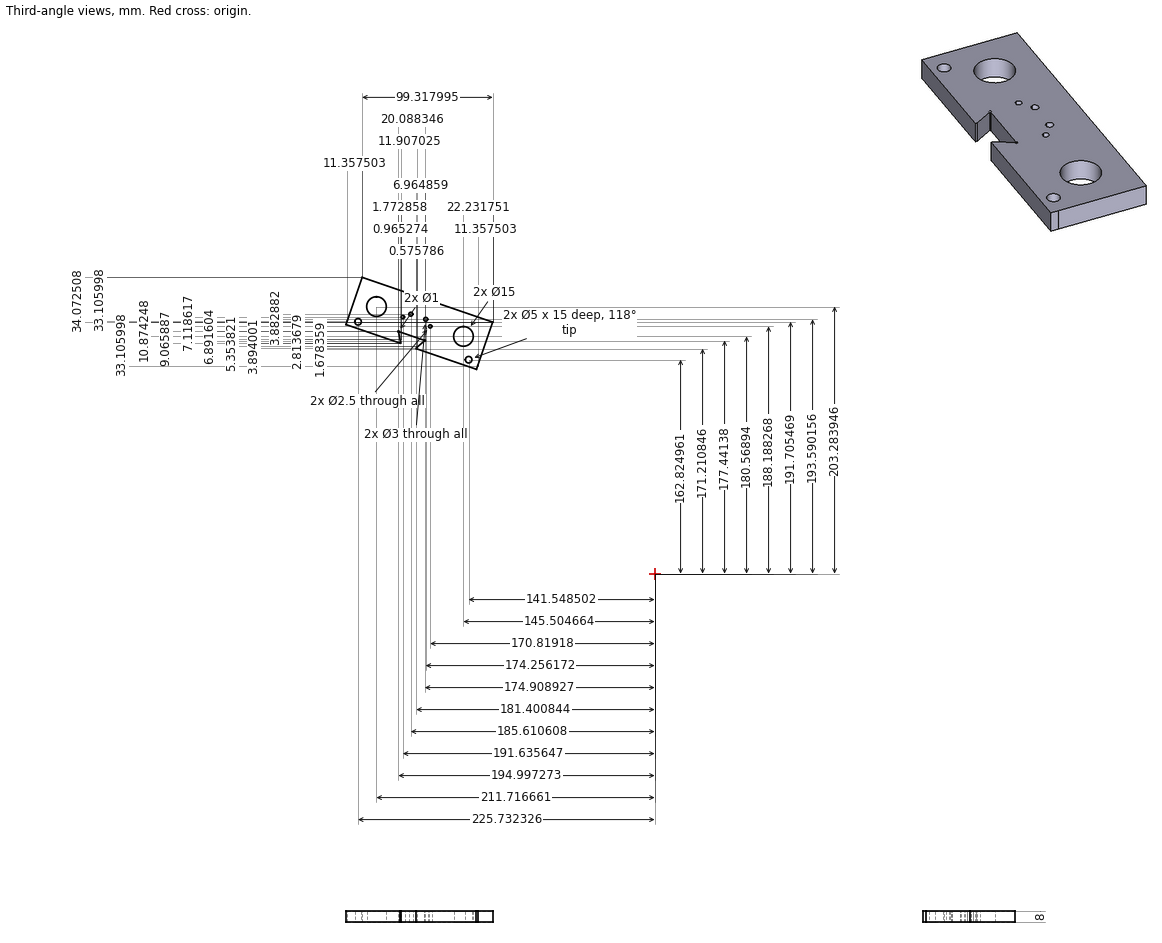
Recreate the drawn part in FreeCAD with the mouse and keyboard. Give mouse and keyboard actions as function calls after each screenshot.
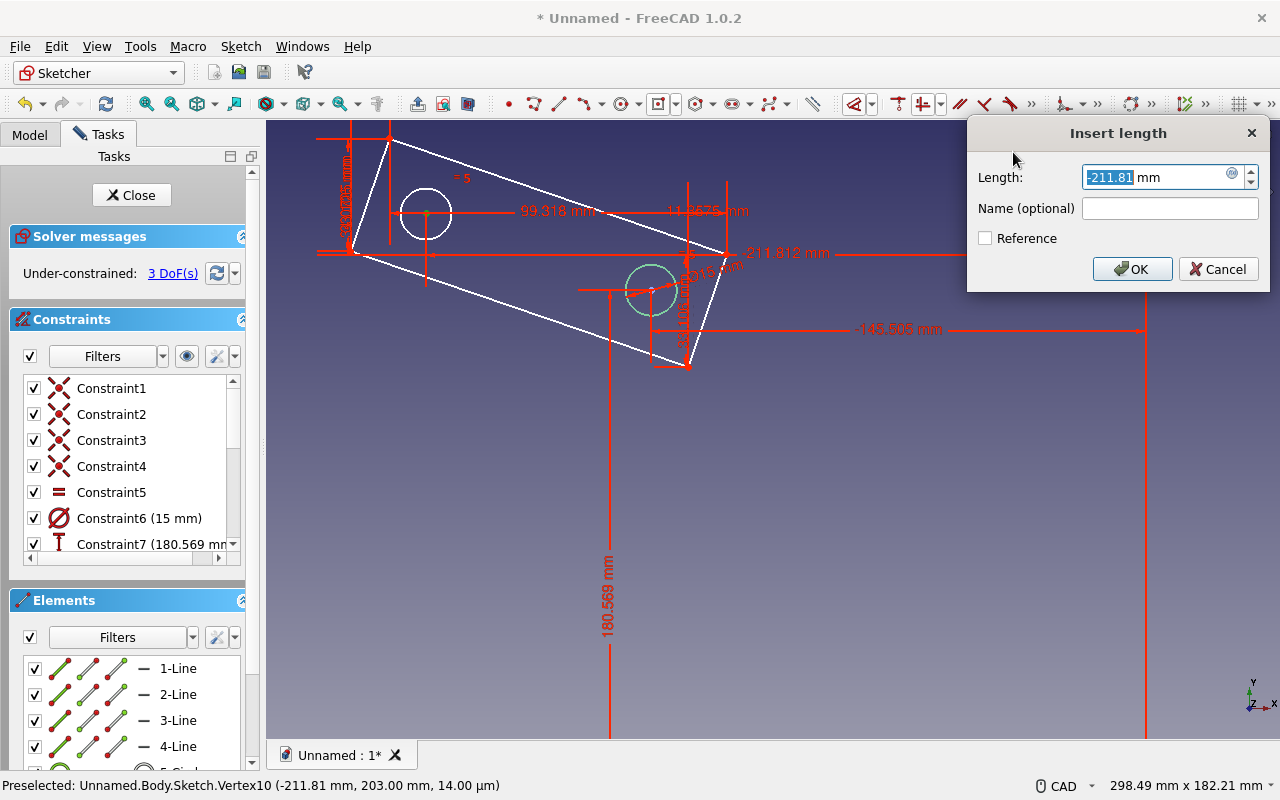
text(-211.716661)
key(Return)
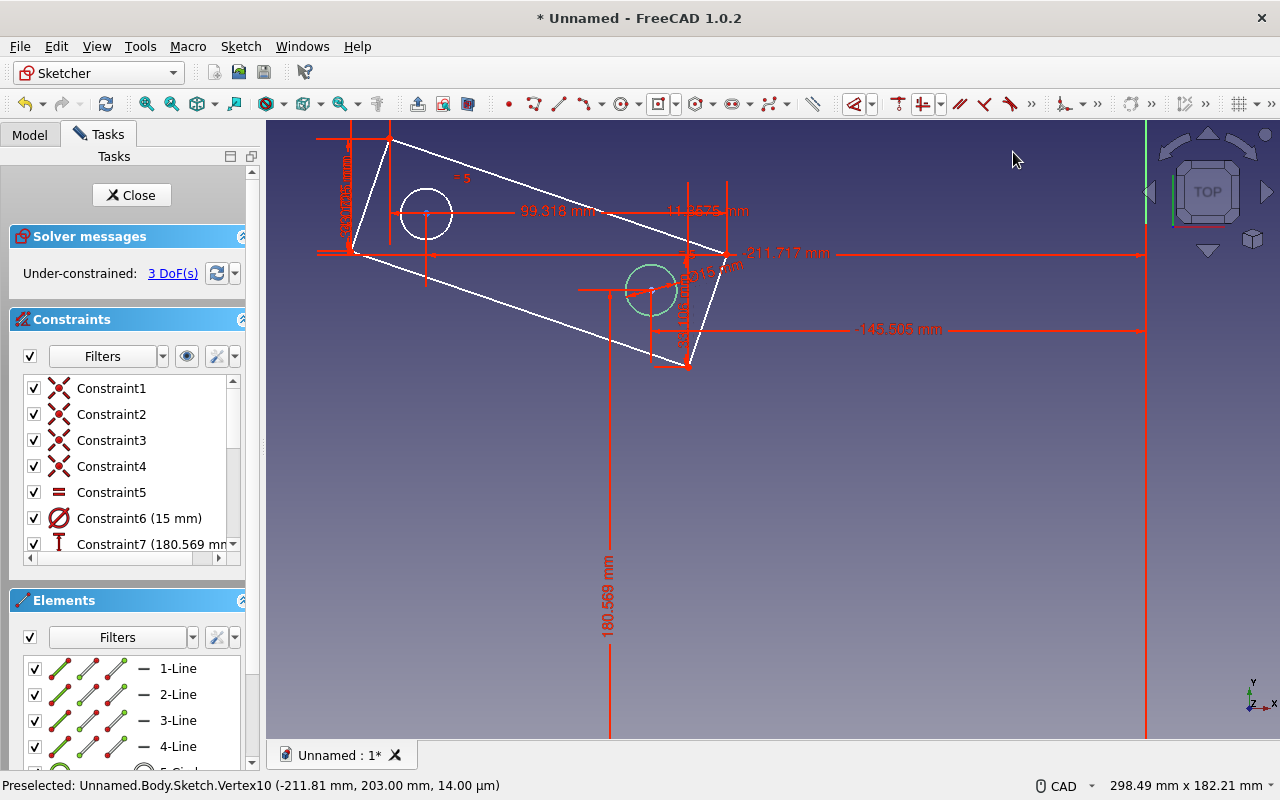
click(426, 214)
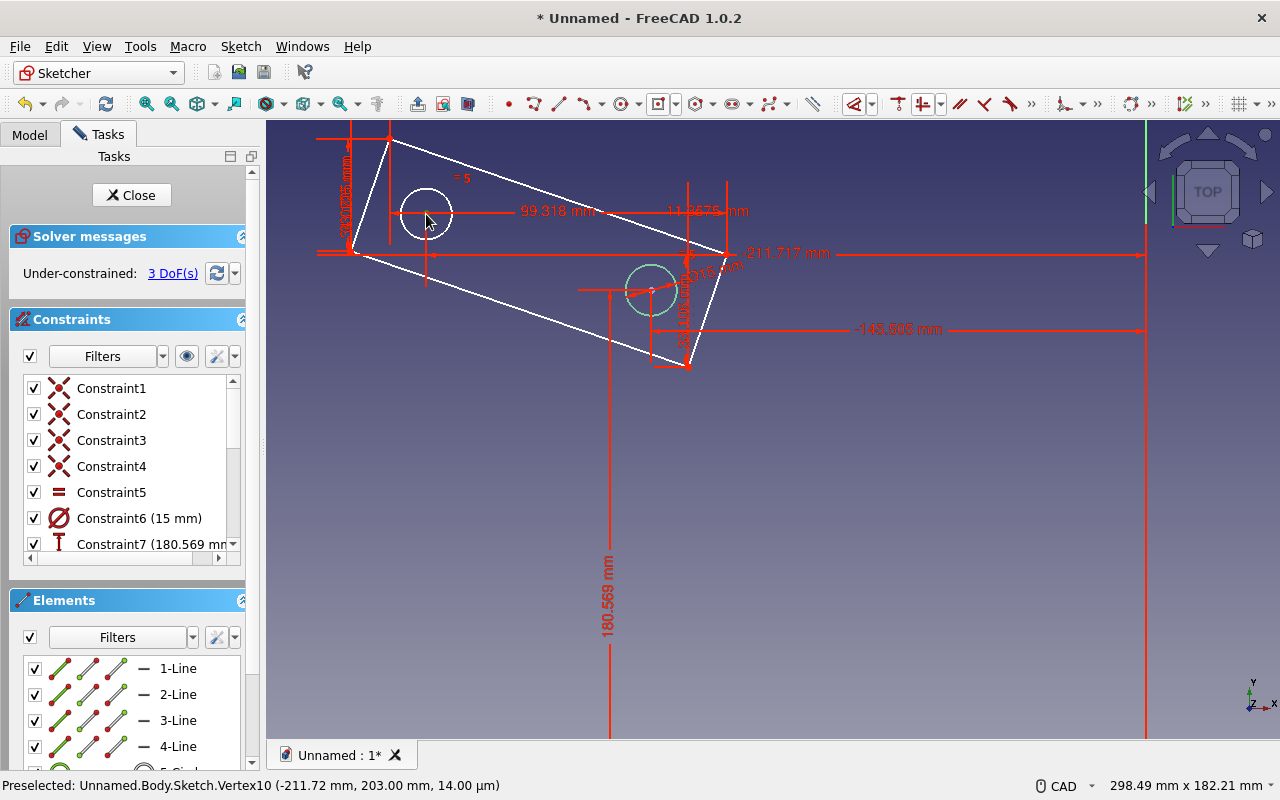
key(i)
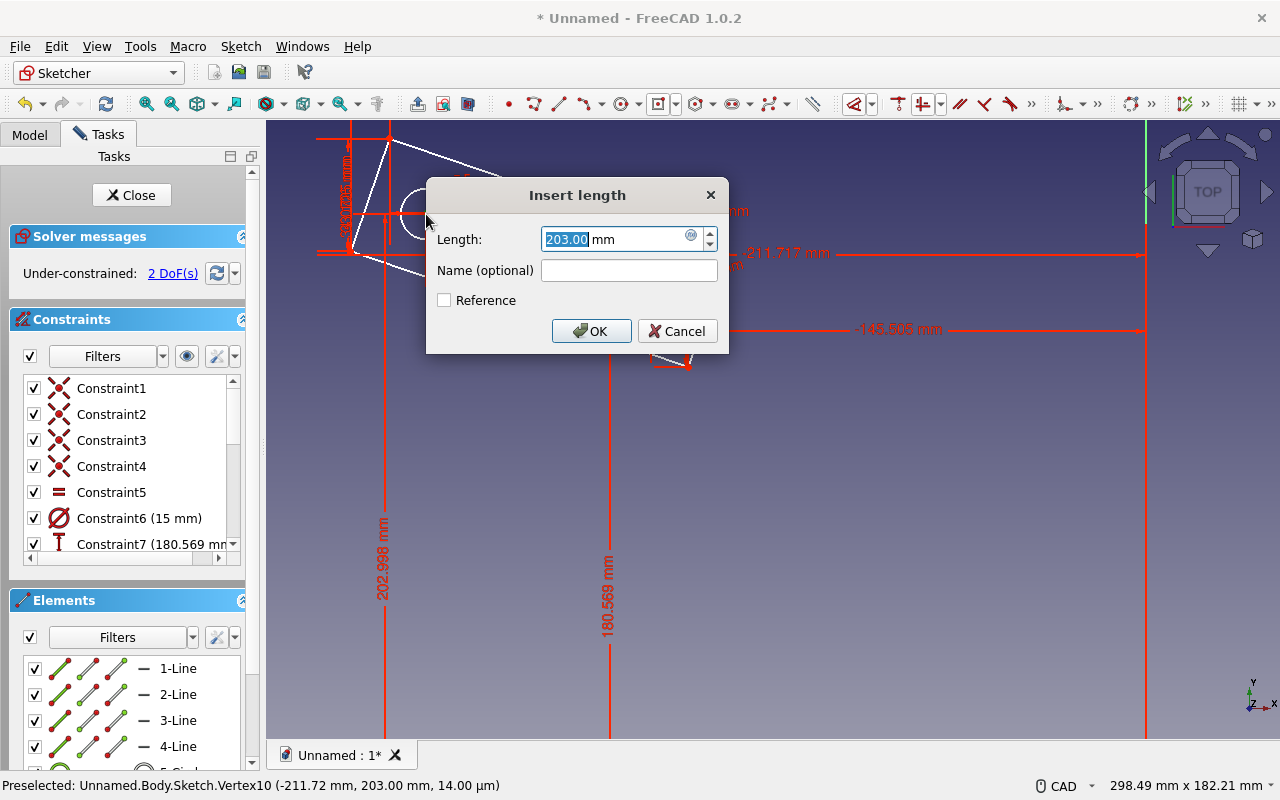
text(203.283946)
key(Return)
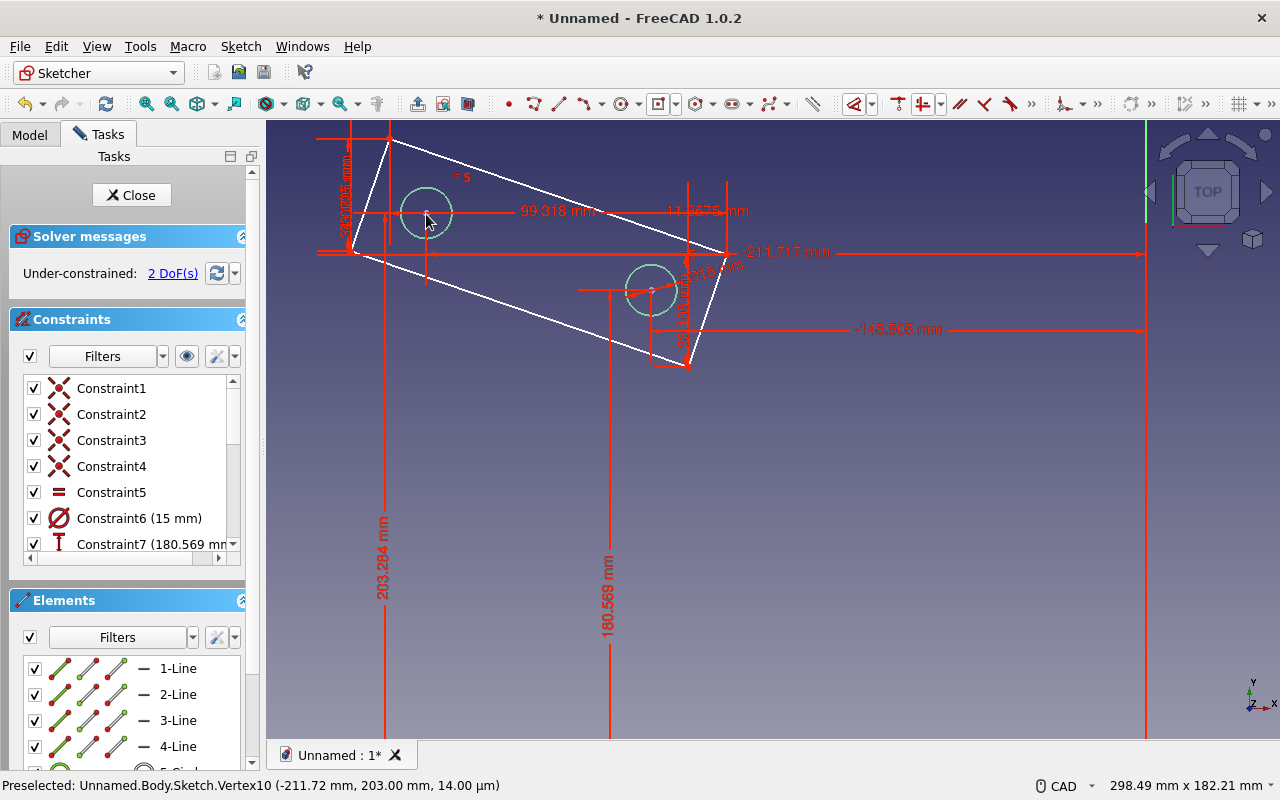
click(727, 255)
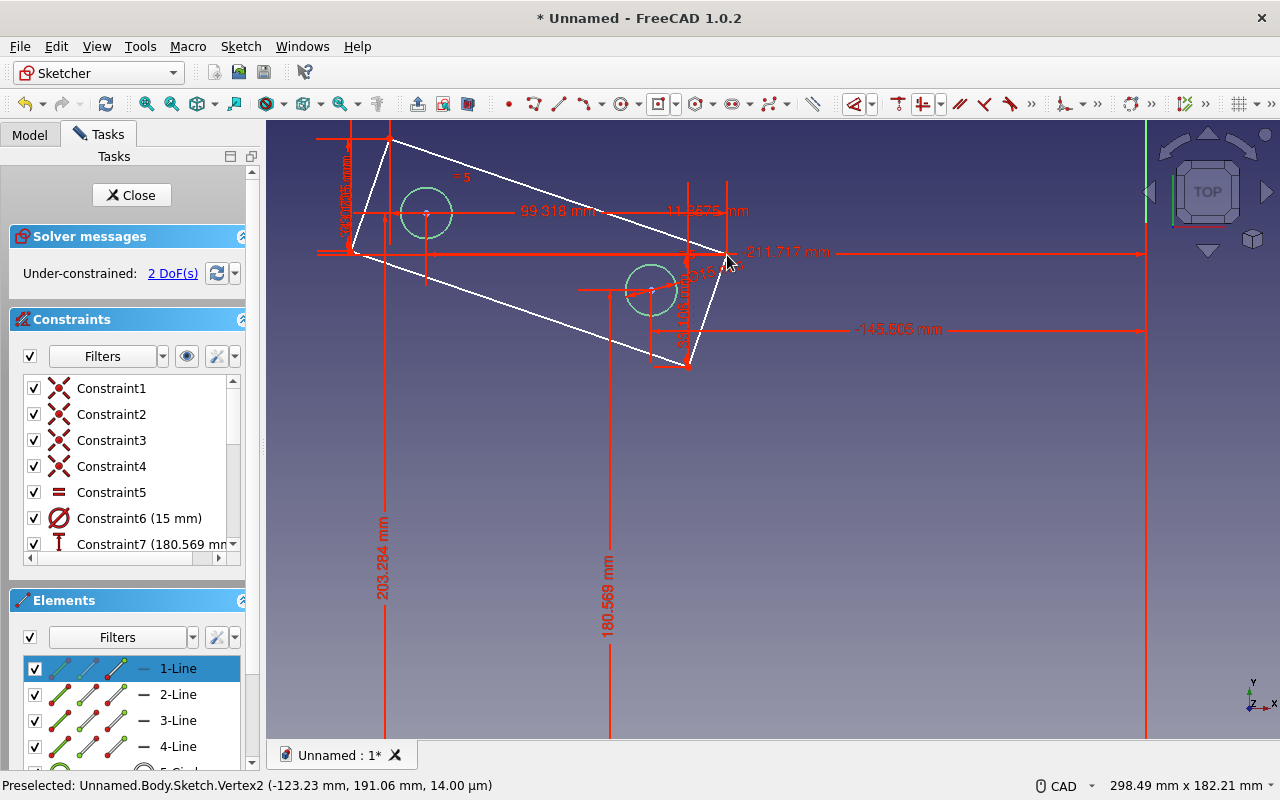
click(651, 290)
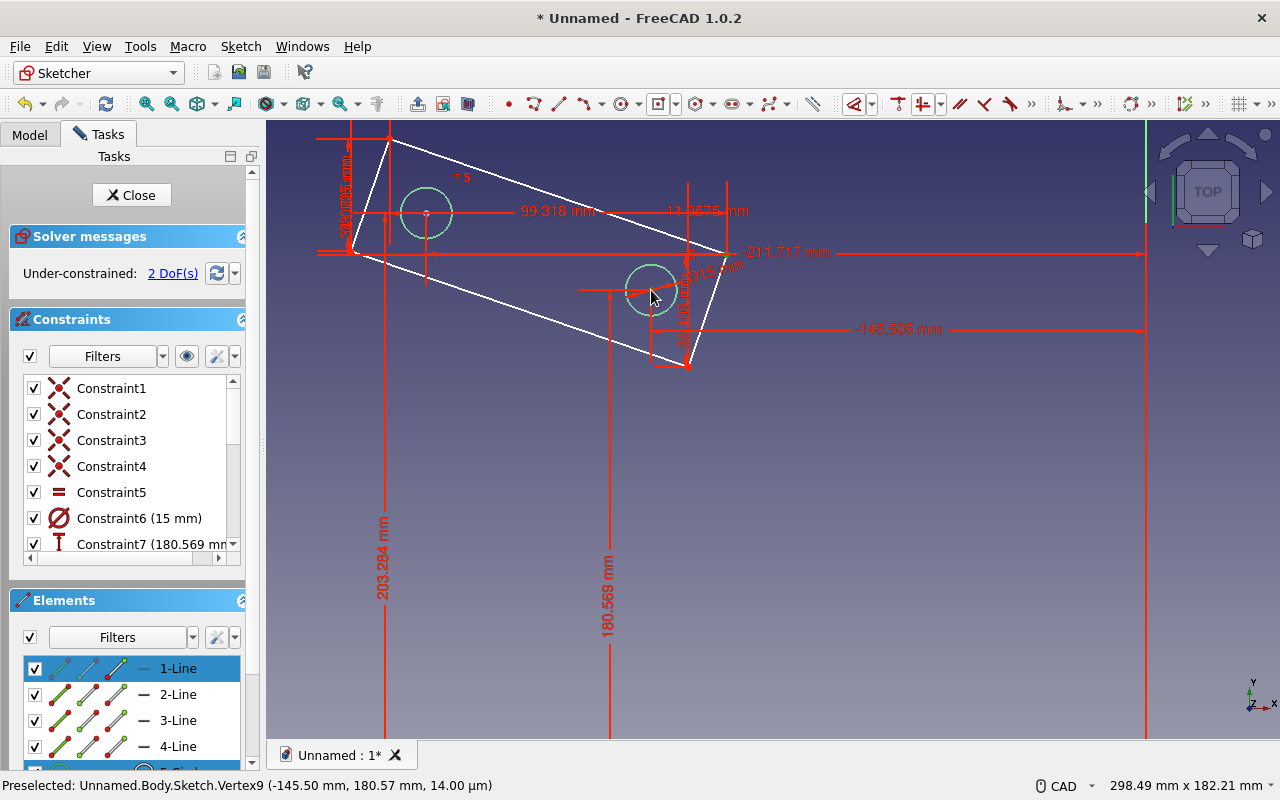
key(l)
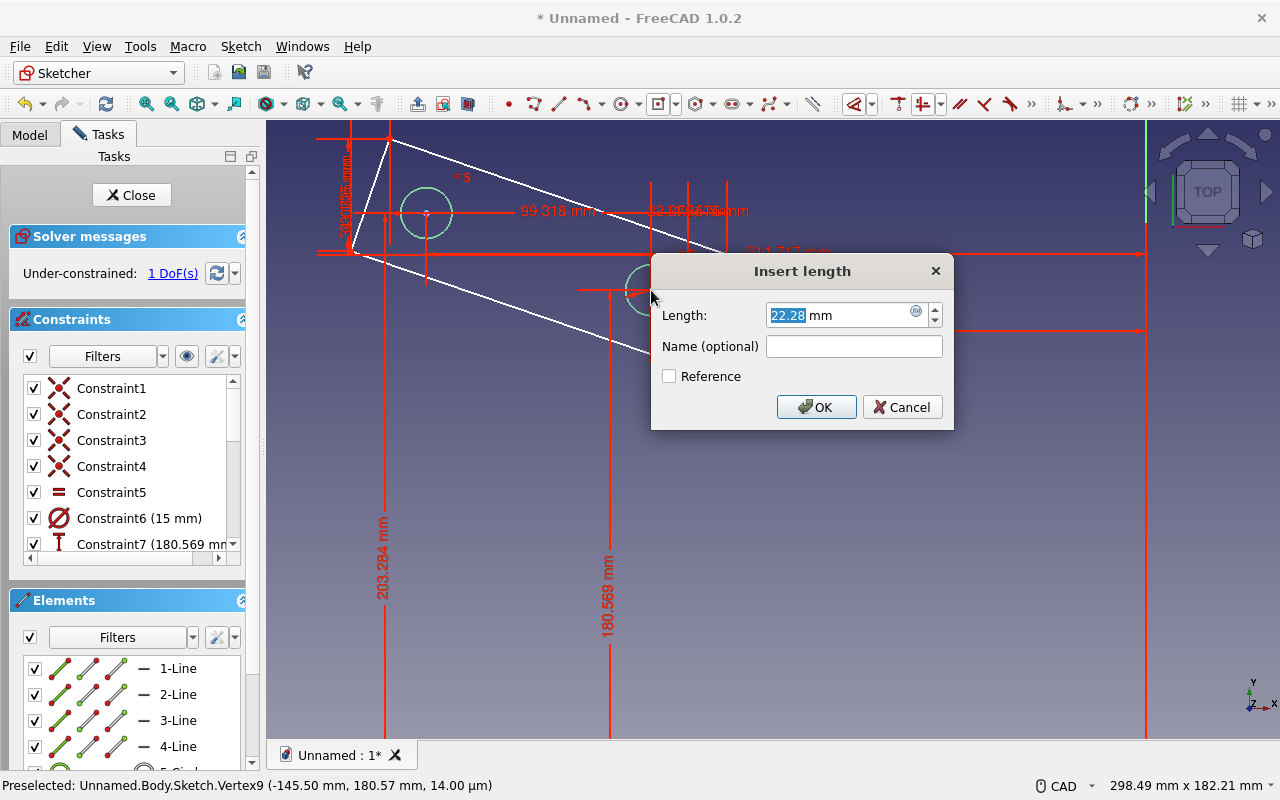
text(22.231751)
key(Return)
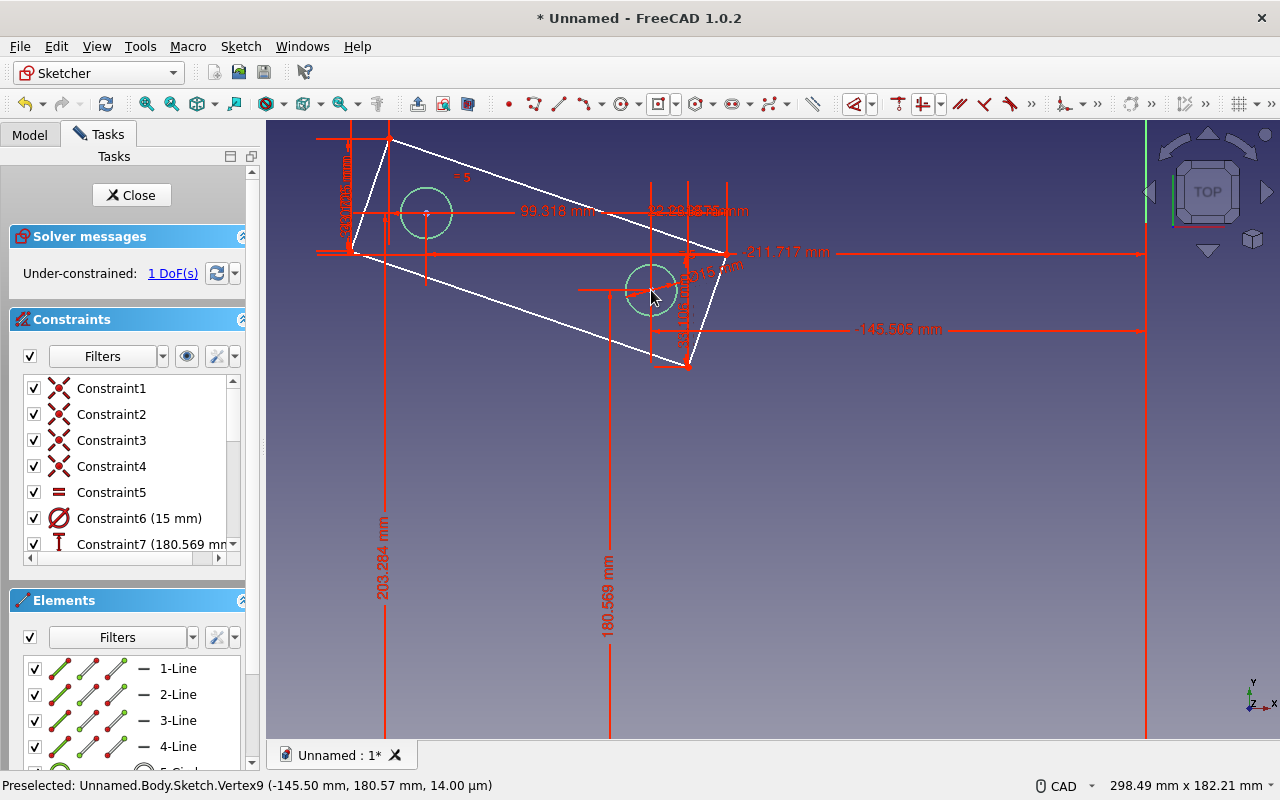
click(727, 255)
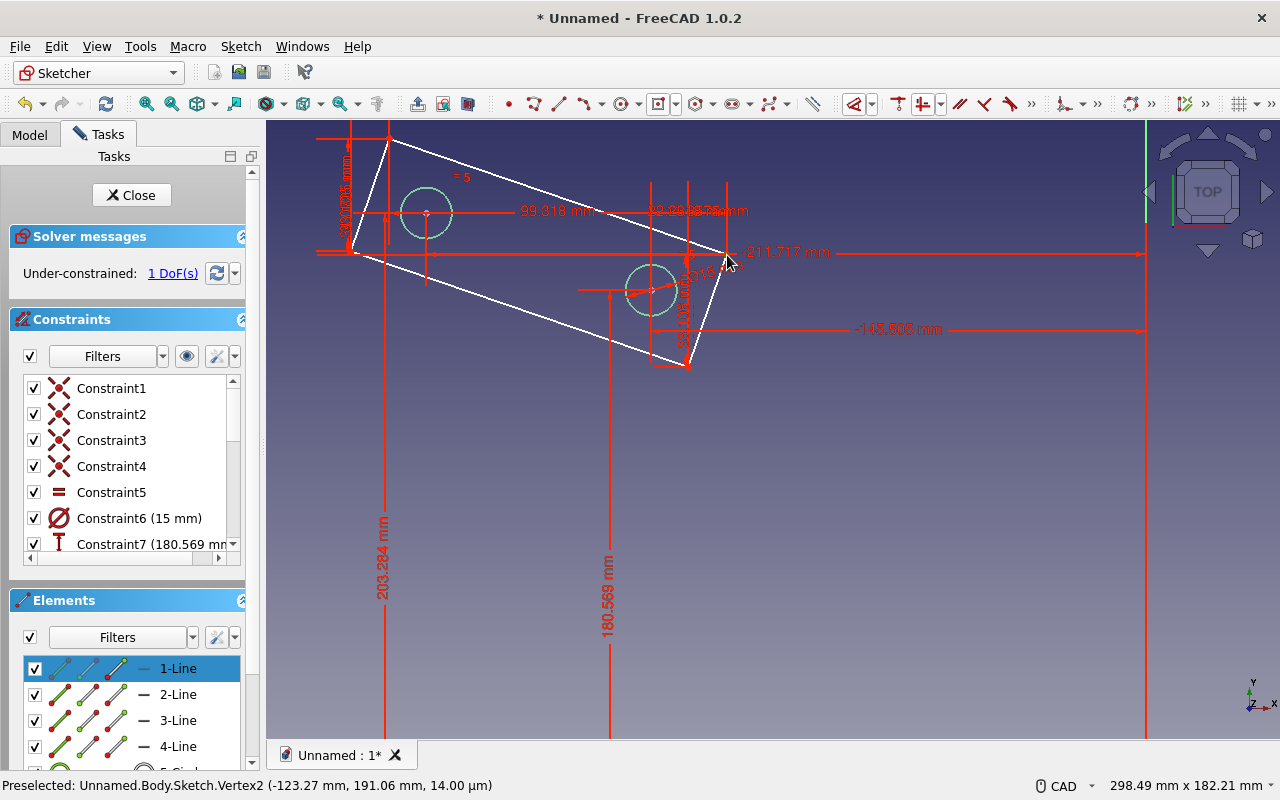
click(651, 290)